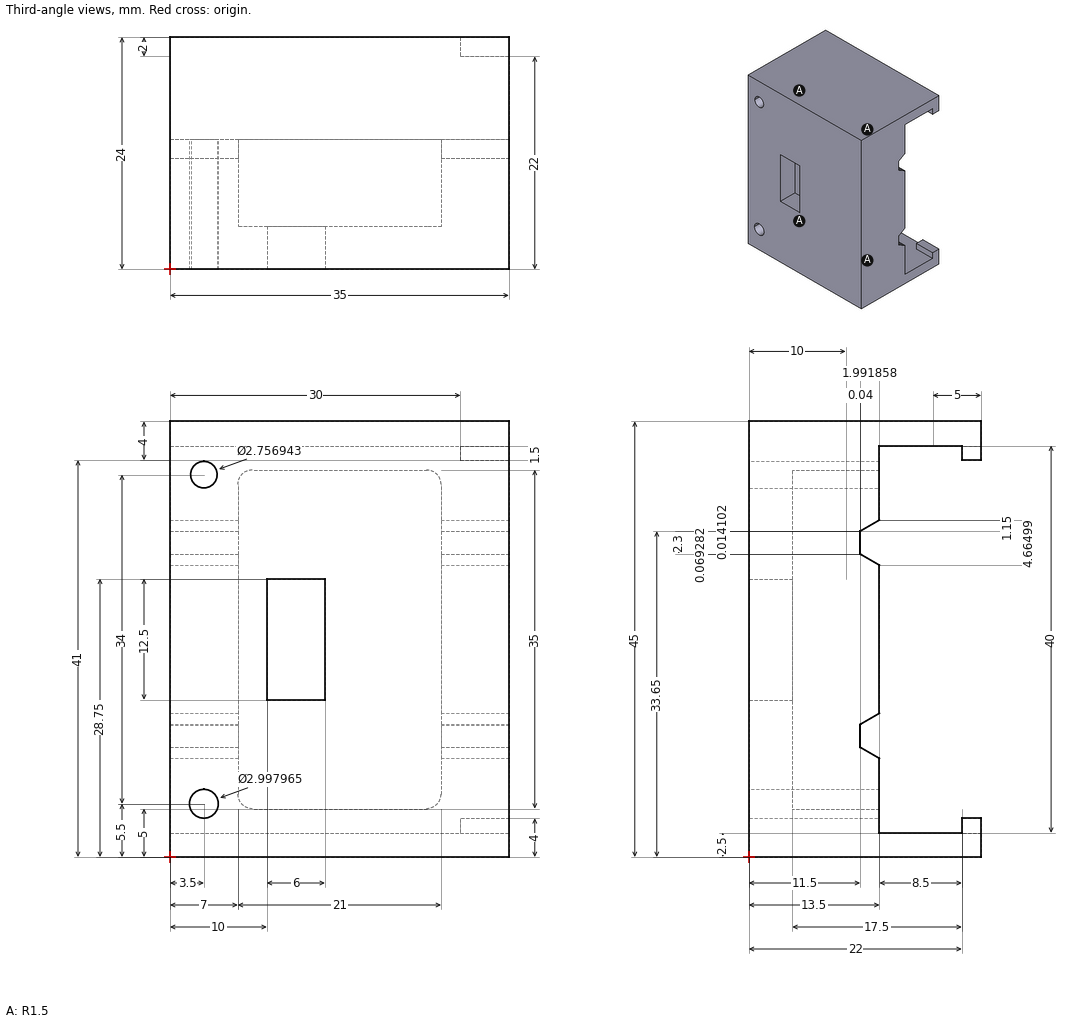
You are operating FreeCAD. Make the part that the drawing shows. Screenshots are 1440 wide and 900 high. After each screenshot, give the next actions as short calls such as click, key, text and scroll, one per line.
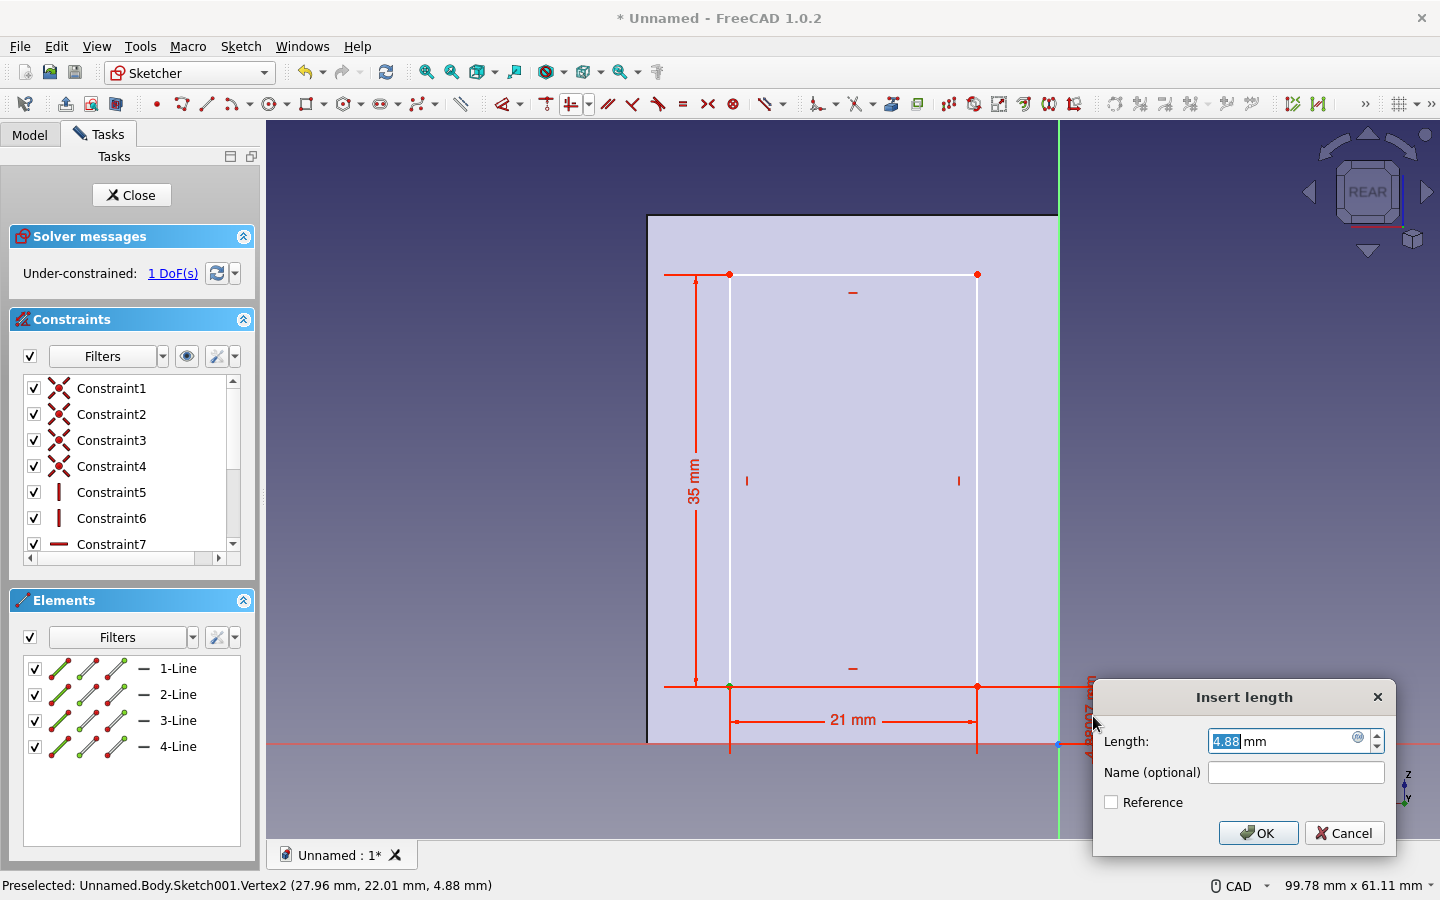
text(5)
key(Return)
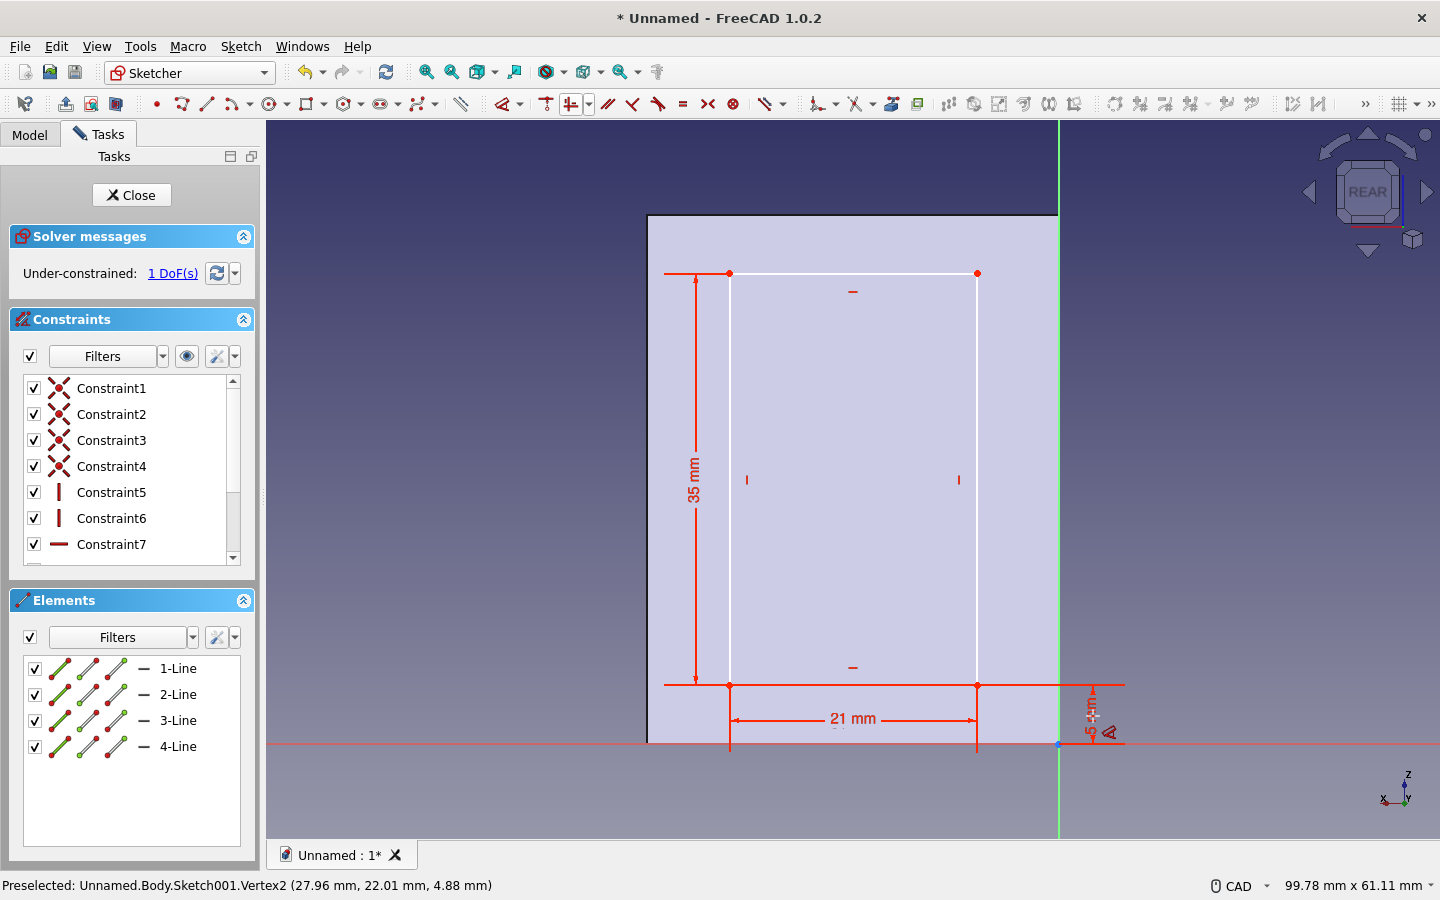
click(977, 685)
click(1018, 778)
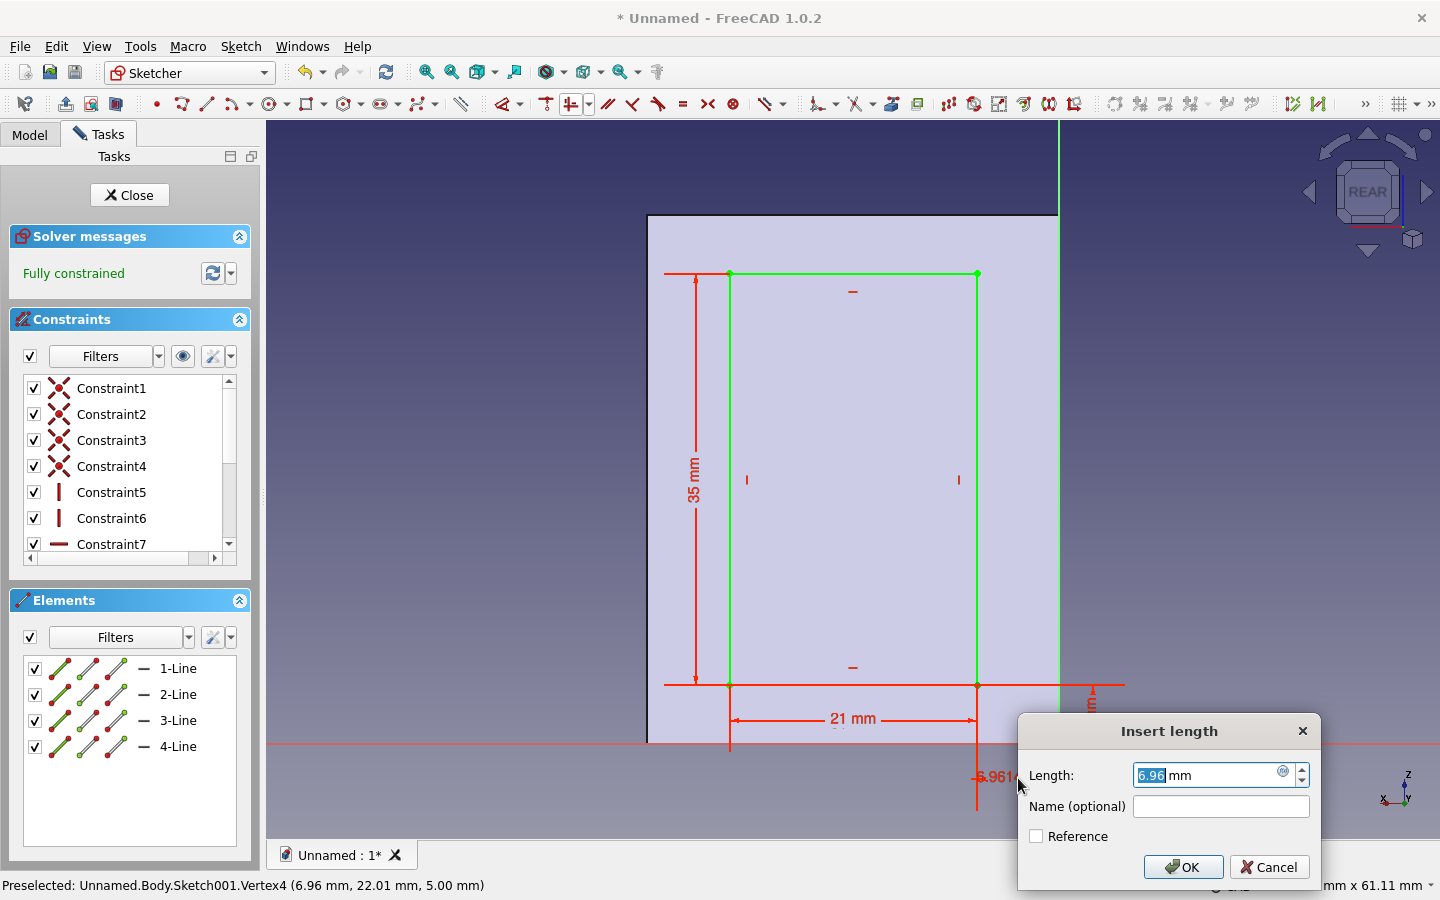
text(7)
key(Return)
key(Escape)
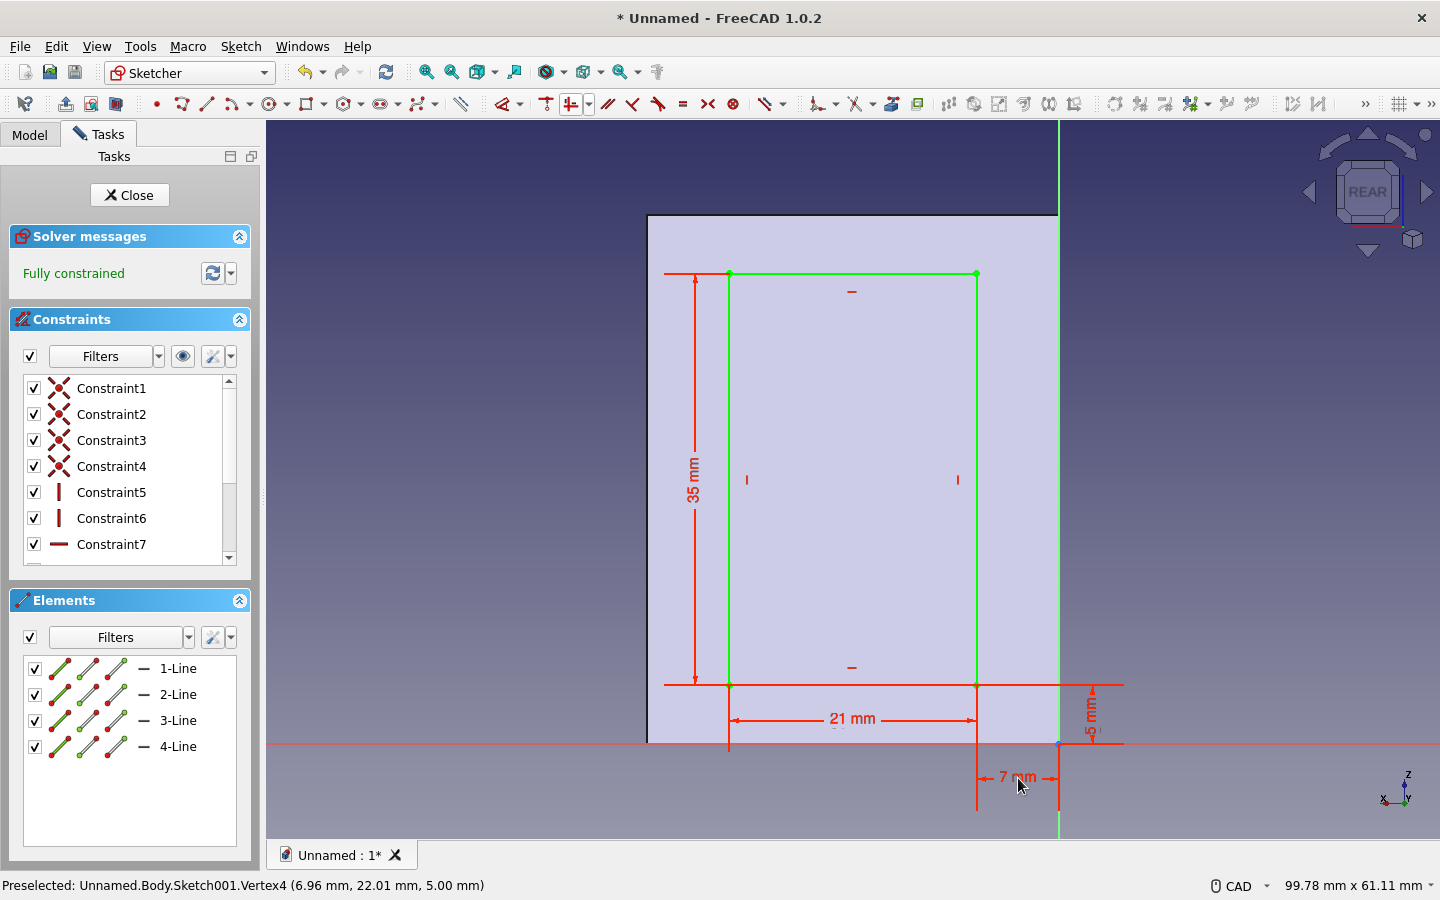
click(130, 195)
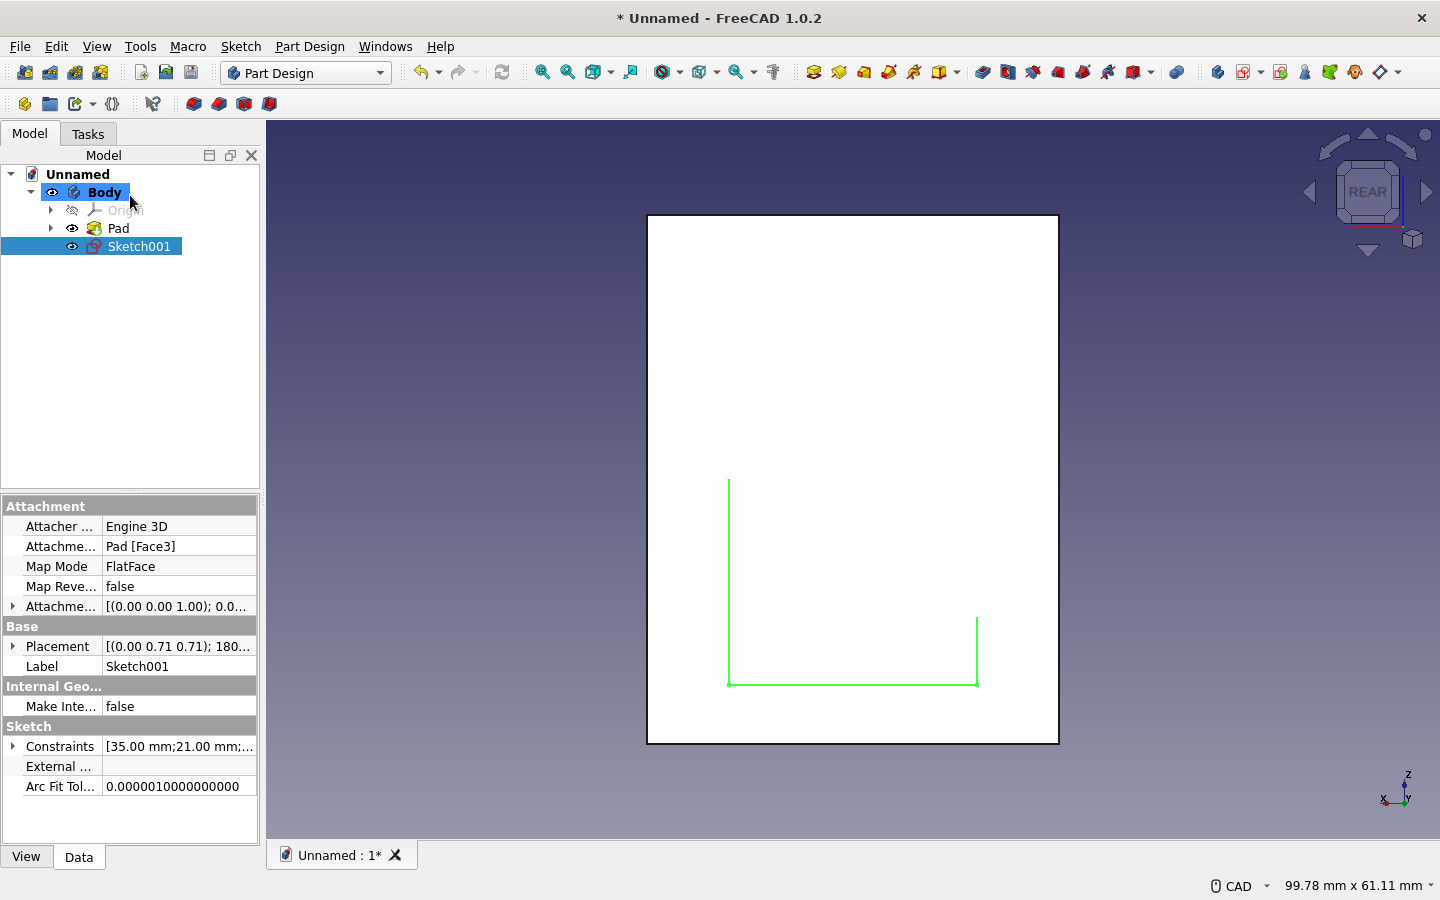
click(983, 72)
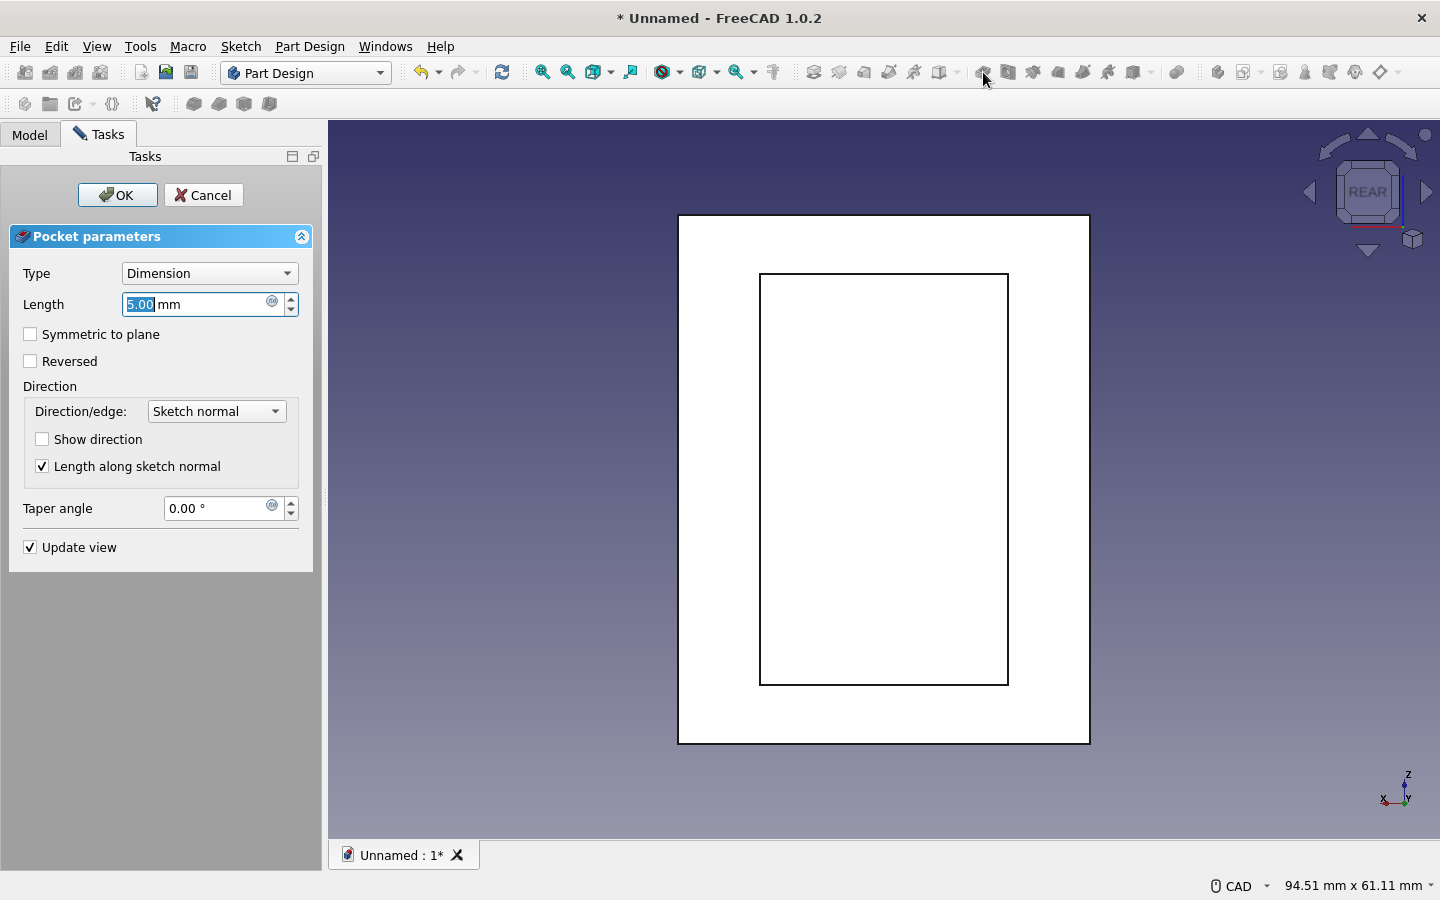
text(17.5)
key(Tab)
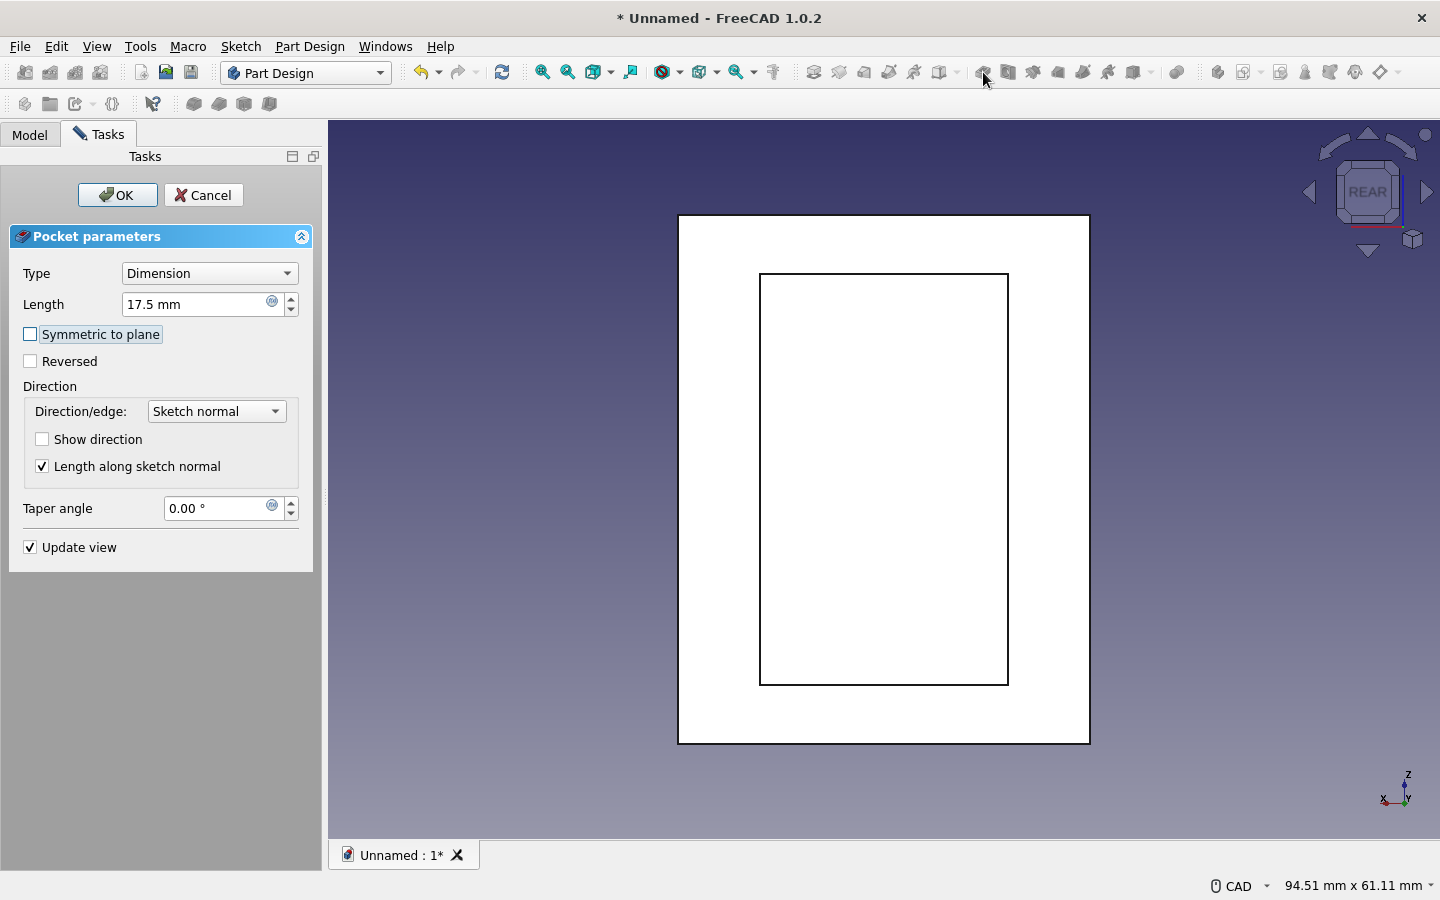
click(118, 195)